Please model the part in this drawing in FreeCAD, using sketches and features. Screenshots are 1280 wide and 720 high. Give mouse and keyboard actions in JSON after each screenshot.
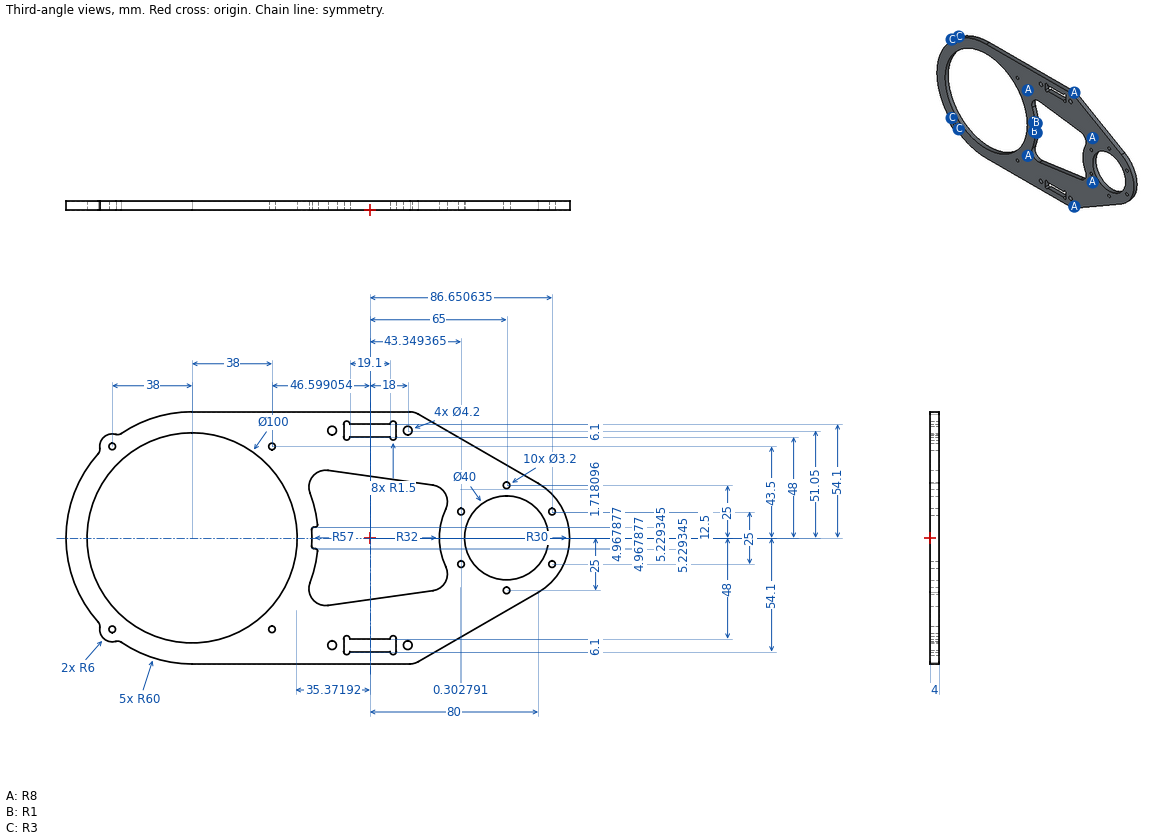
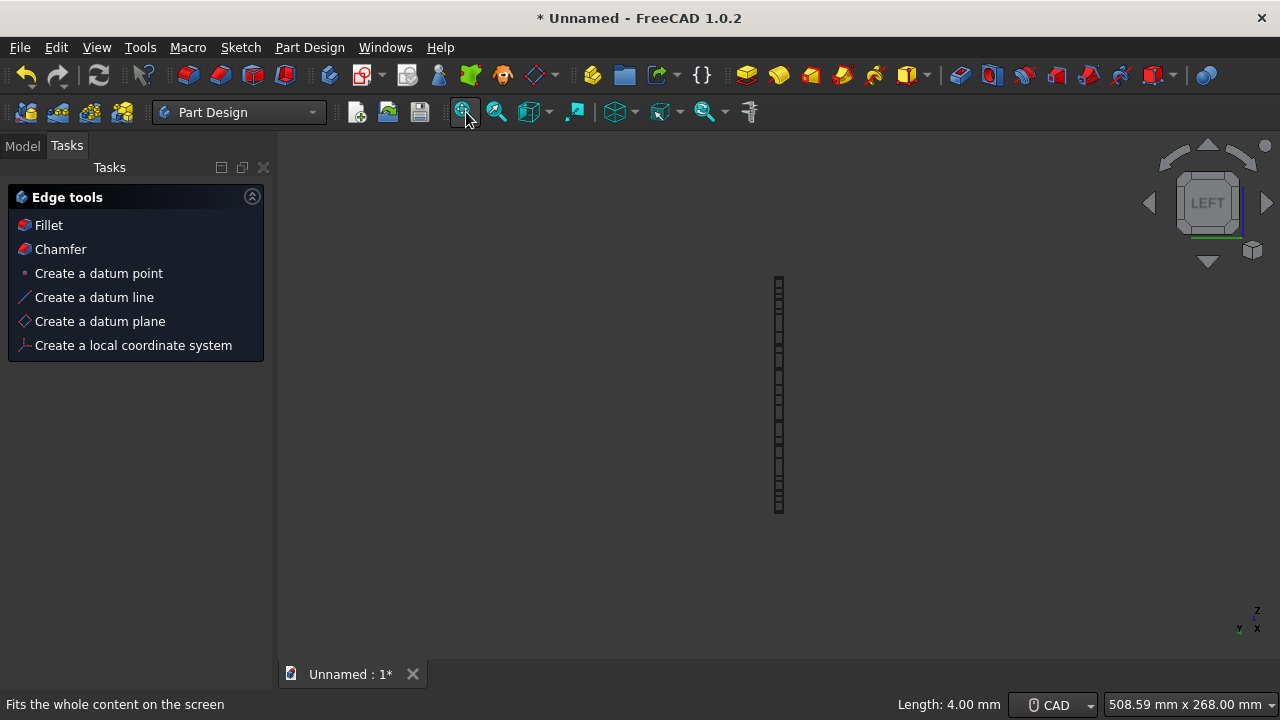
{"action": "key", "text": "0"}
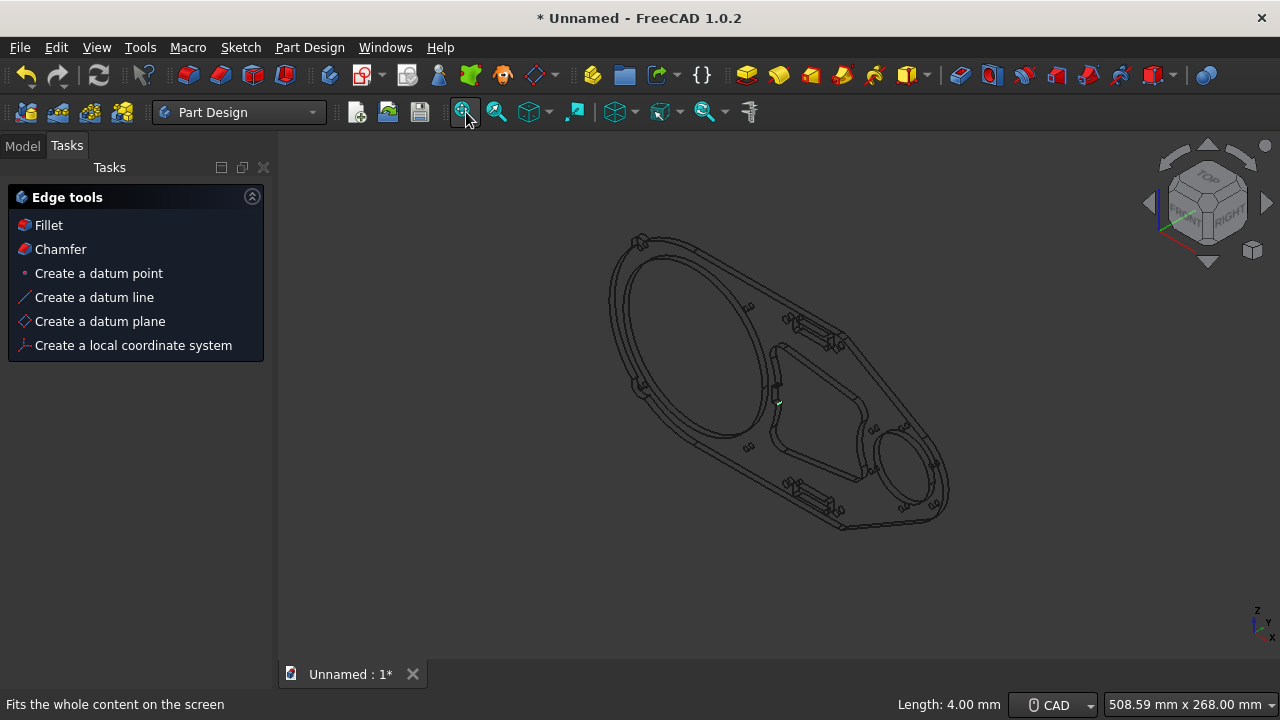
{"action": "scroll", "coordinate": [775, 400], "scroll_direction": "up", "scroll_amount": 9}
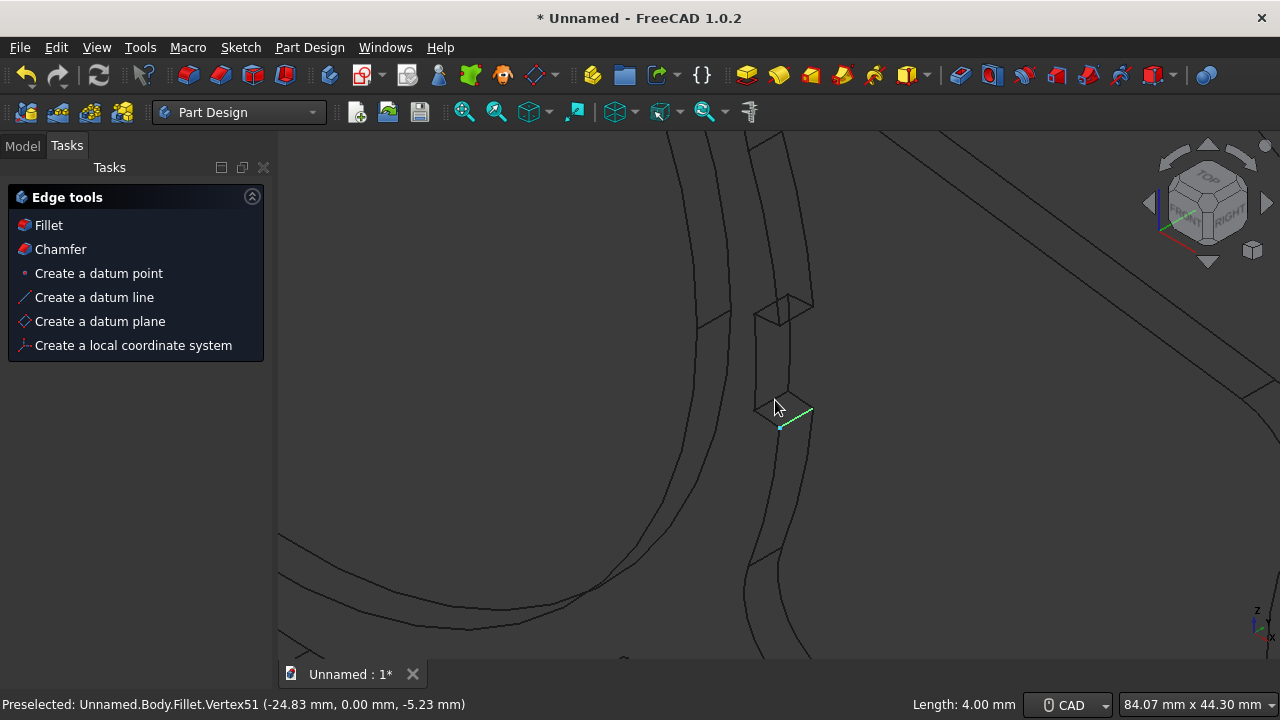
{"action": "left_click", "coordinate": [771, 400], "text": "ctrl"}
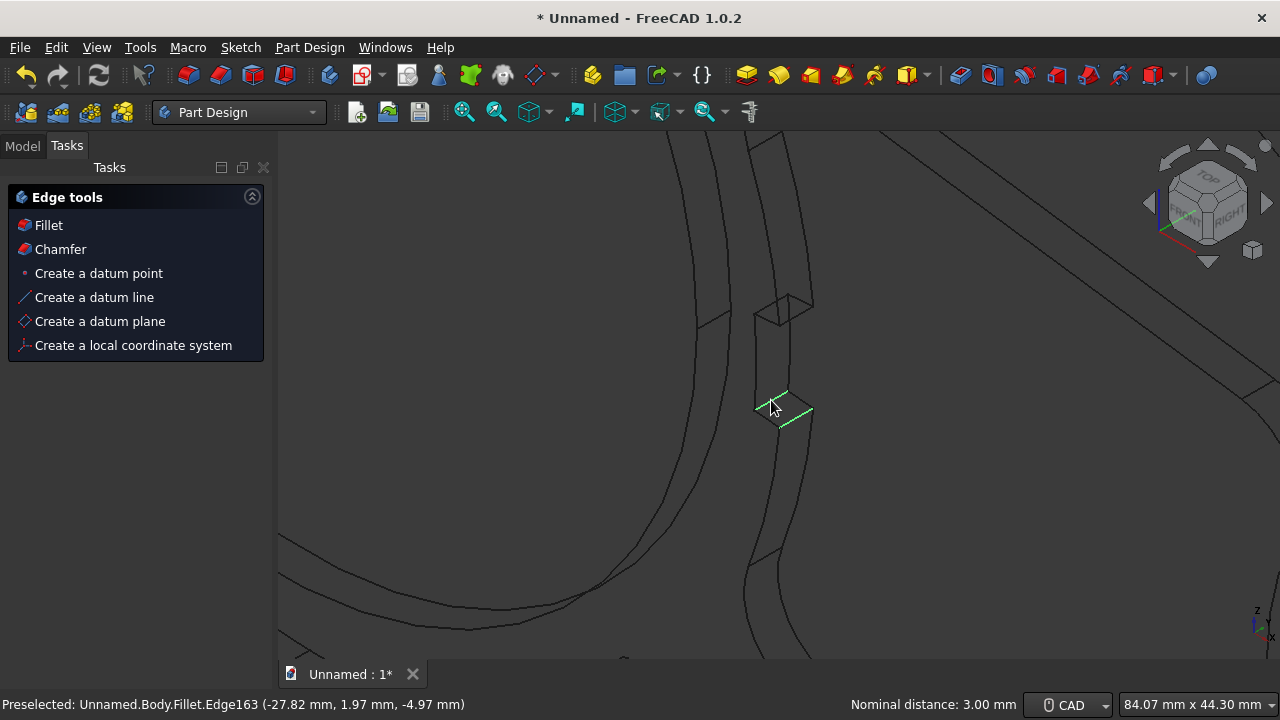
{"action": "left_click", "coordinate": [771, 303], "text": "ctrl"}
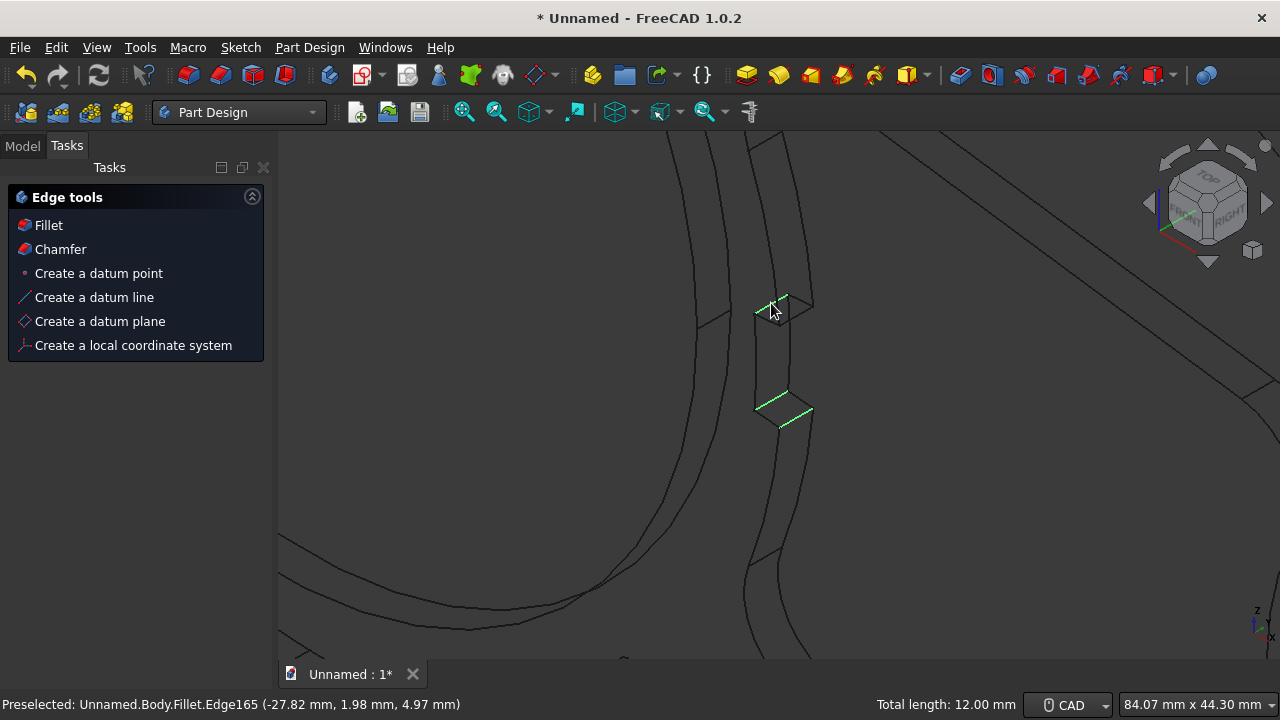
{"action": "left_click", "coordinate": [796, 315], "text": "ctrl"}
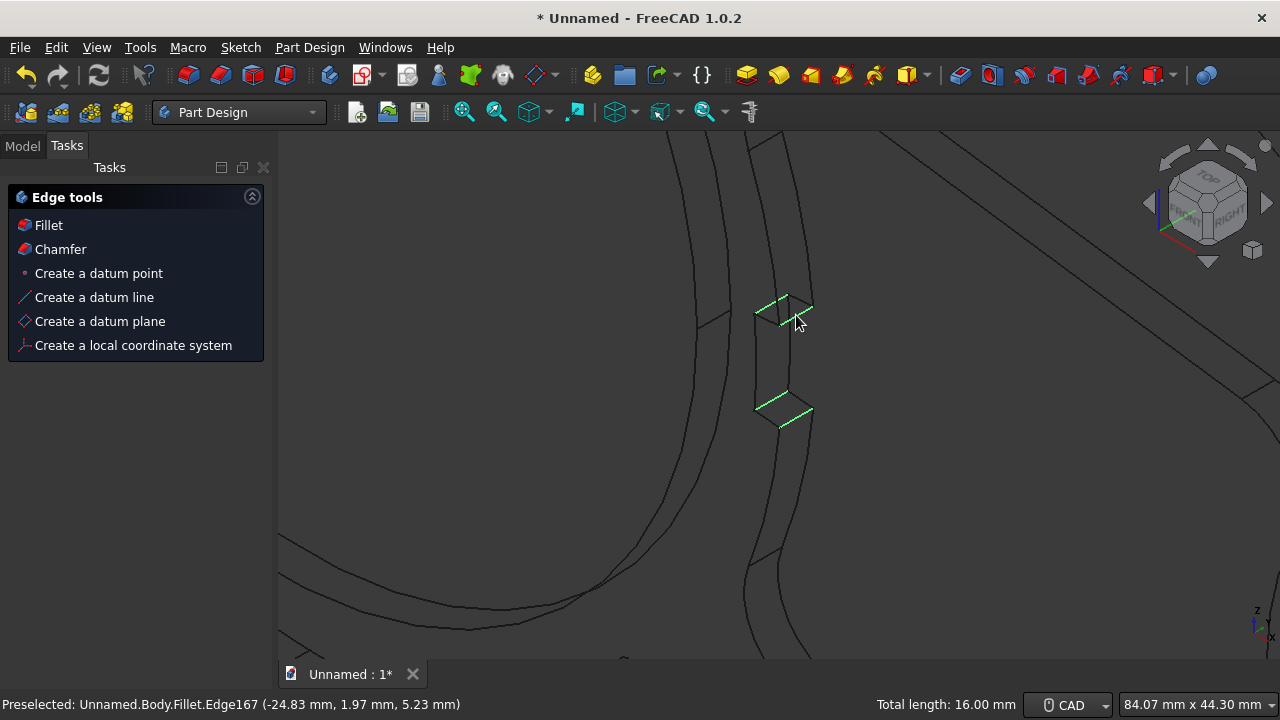
{"action": "key", "text": "v 1"}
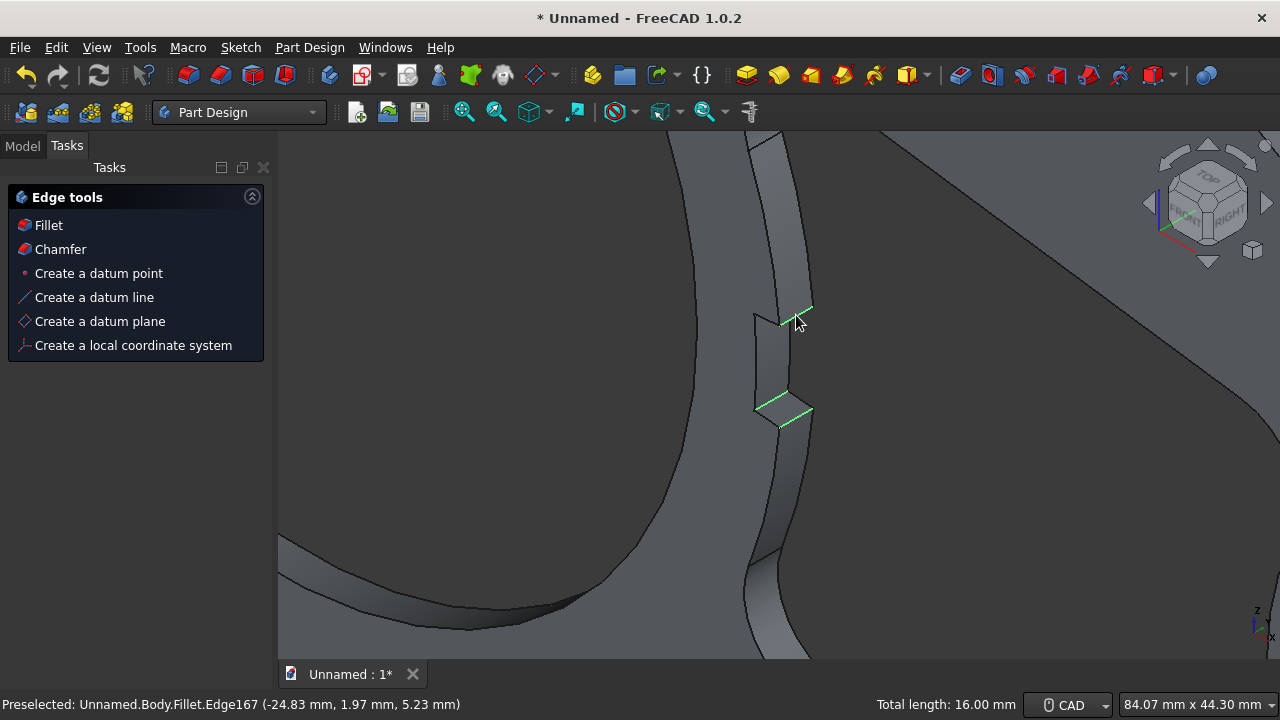
{"action": "left_click", "coordinate": [190, 76]}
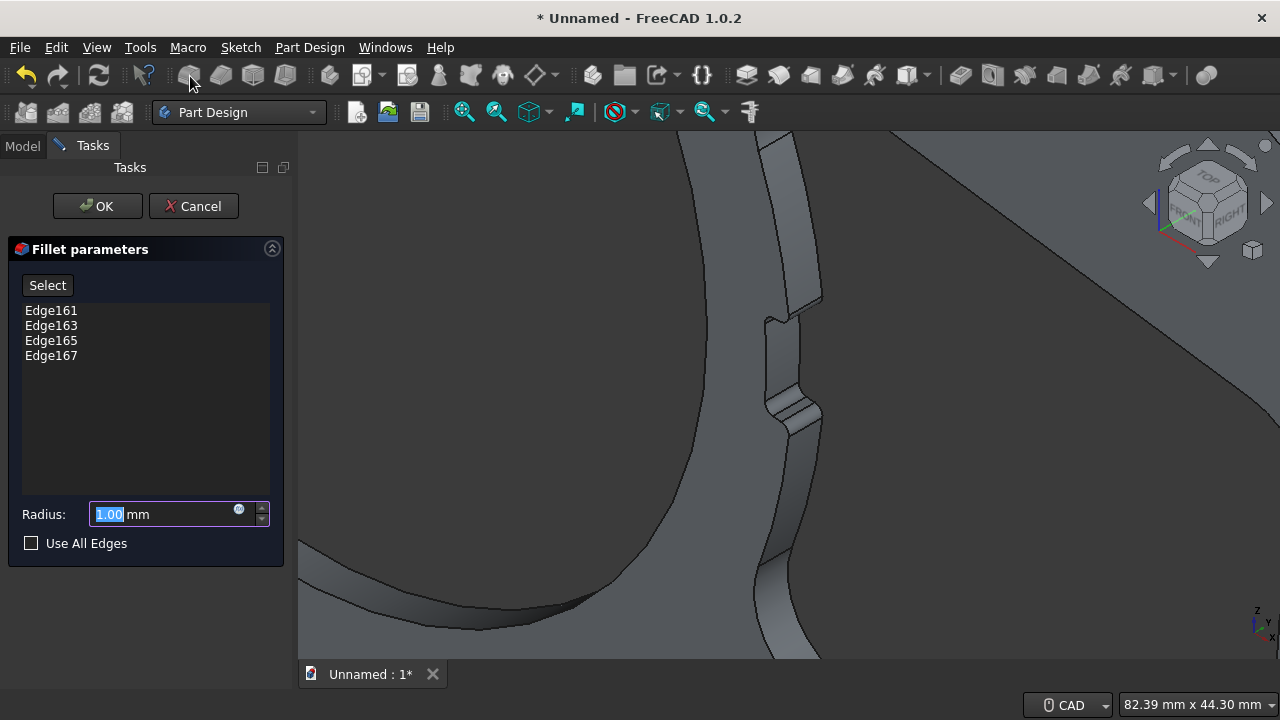
{"action": "type", "text": "1"}
{"action": "key", "text": "Tab"}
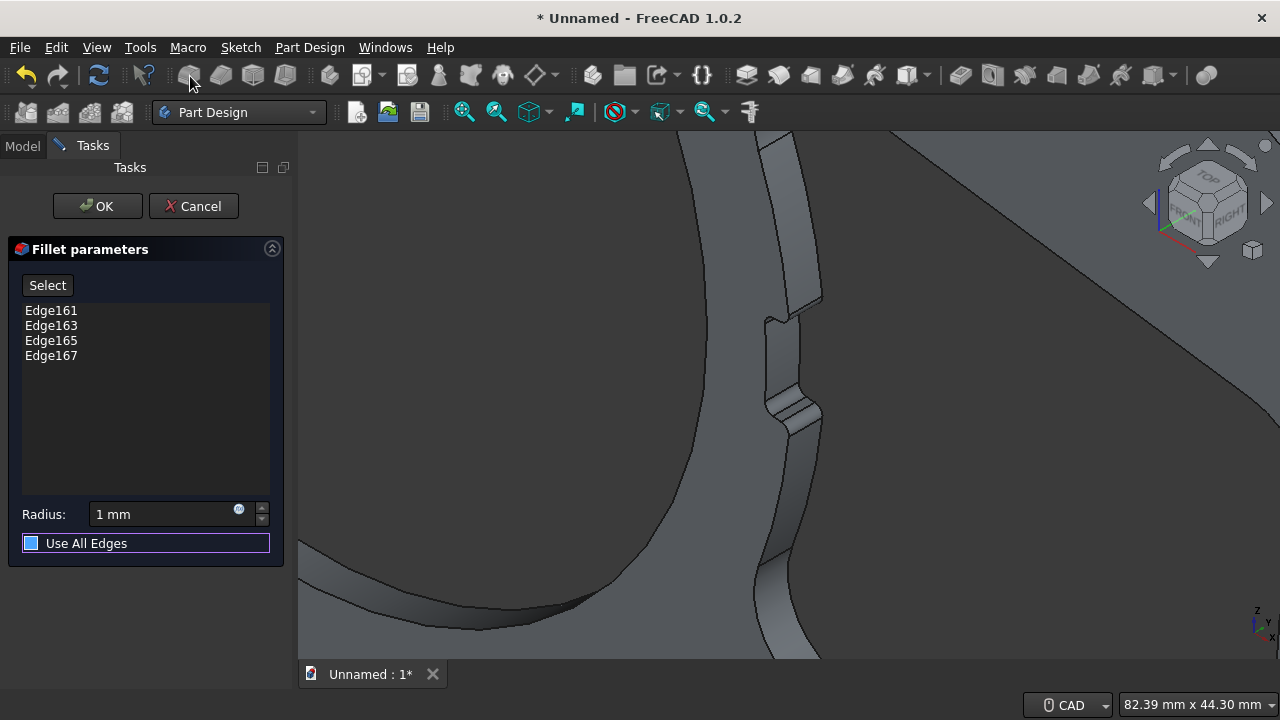
{"action": "left_click", "coordinate": [98, 206]}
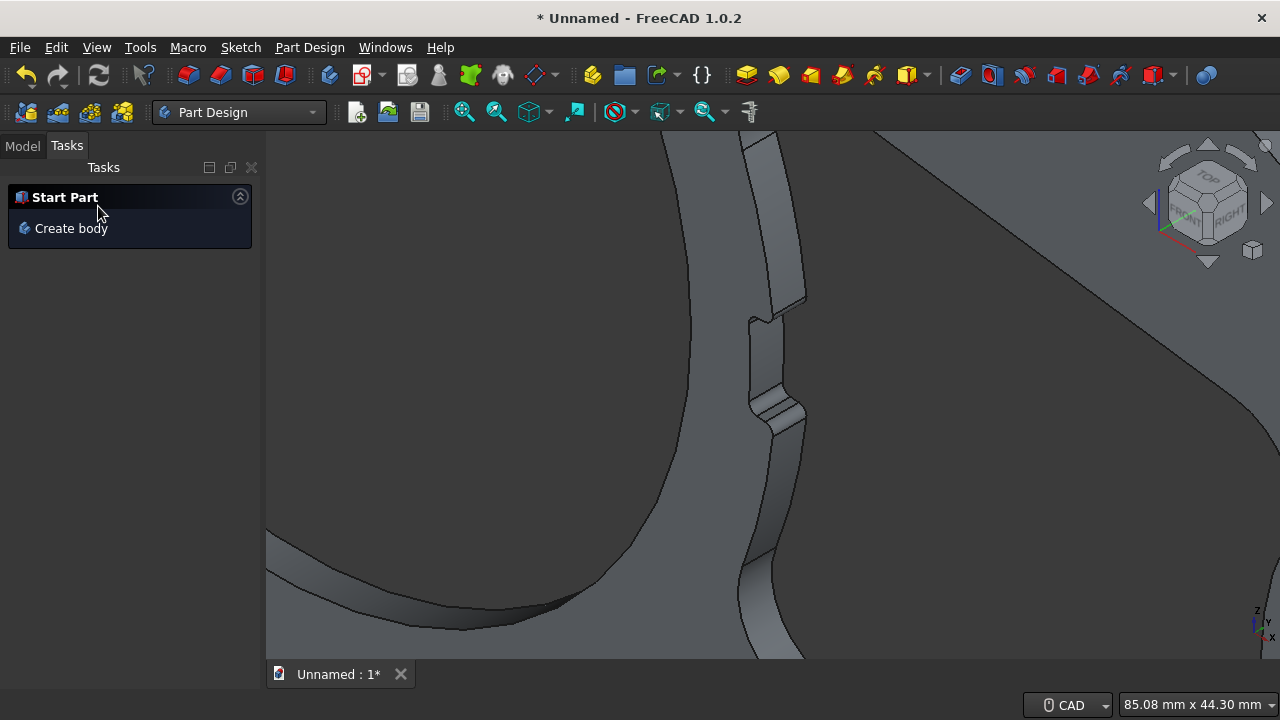
{"action": "left_click", "coordinate": [466, 112]}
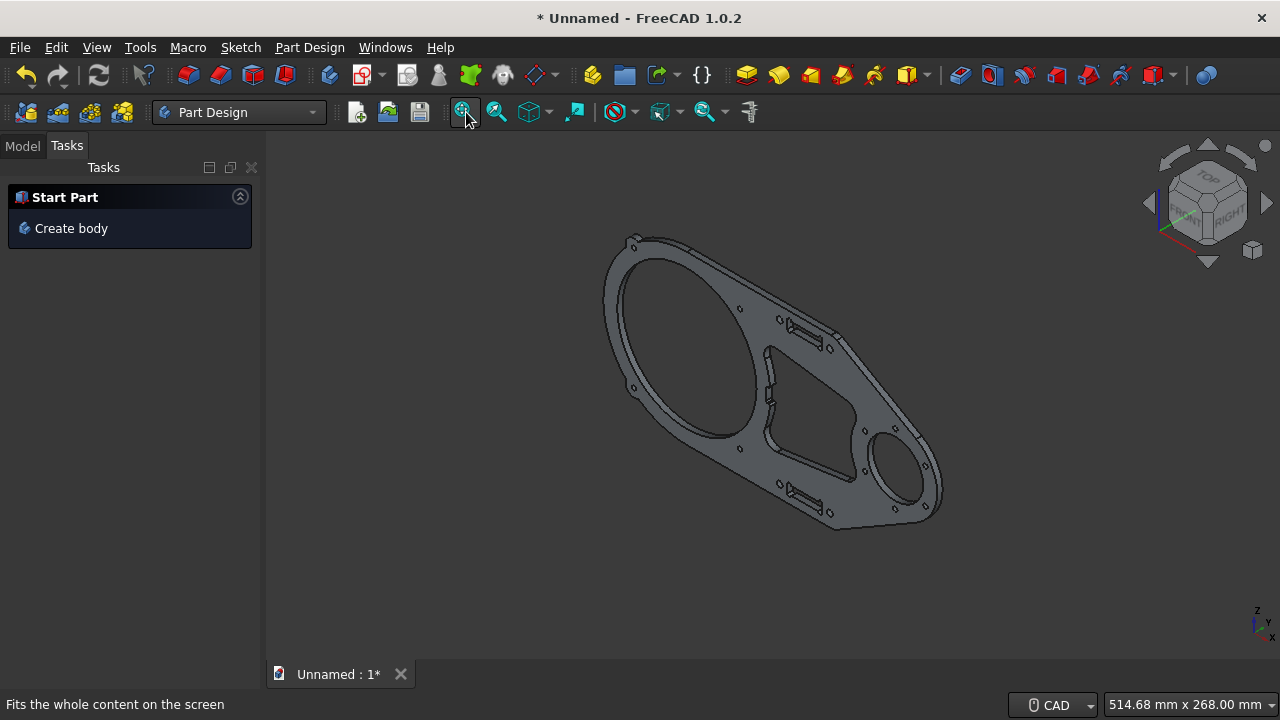
{"action": "scroll", "coordinate": [641, 239], "scroll_direction": "up", "scroll_amount": 9}